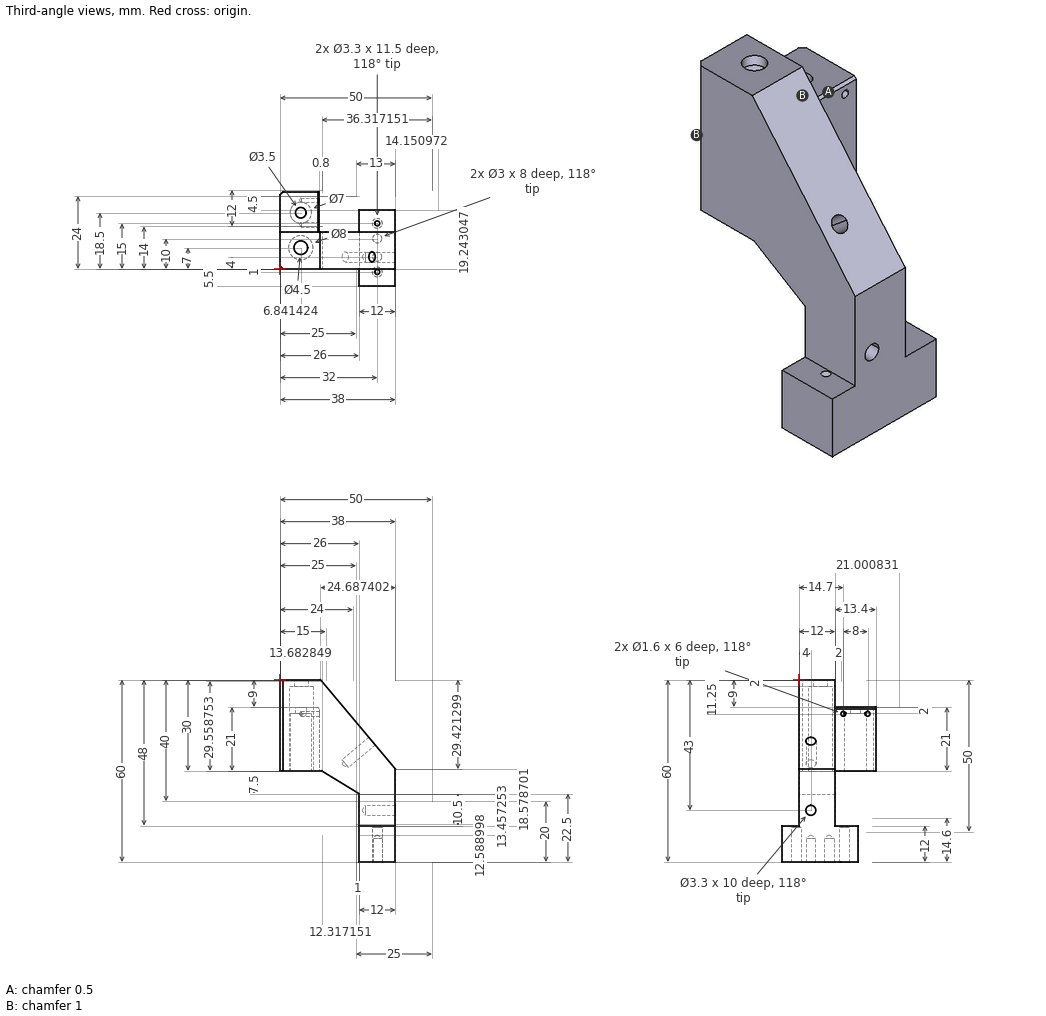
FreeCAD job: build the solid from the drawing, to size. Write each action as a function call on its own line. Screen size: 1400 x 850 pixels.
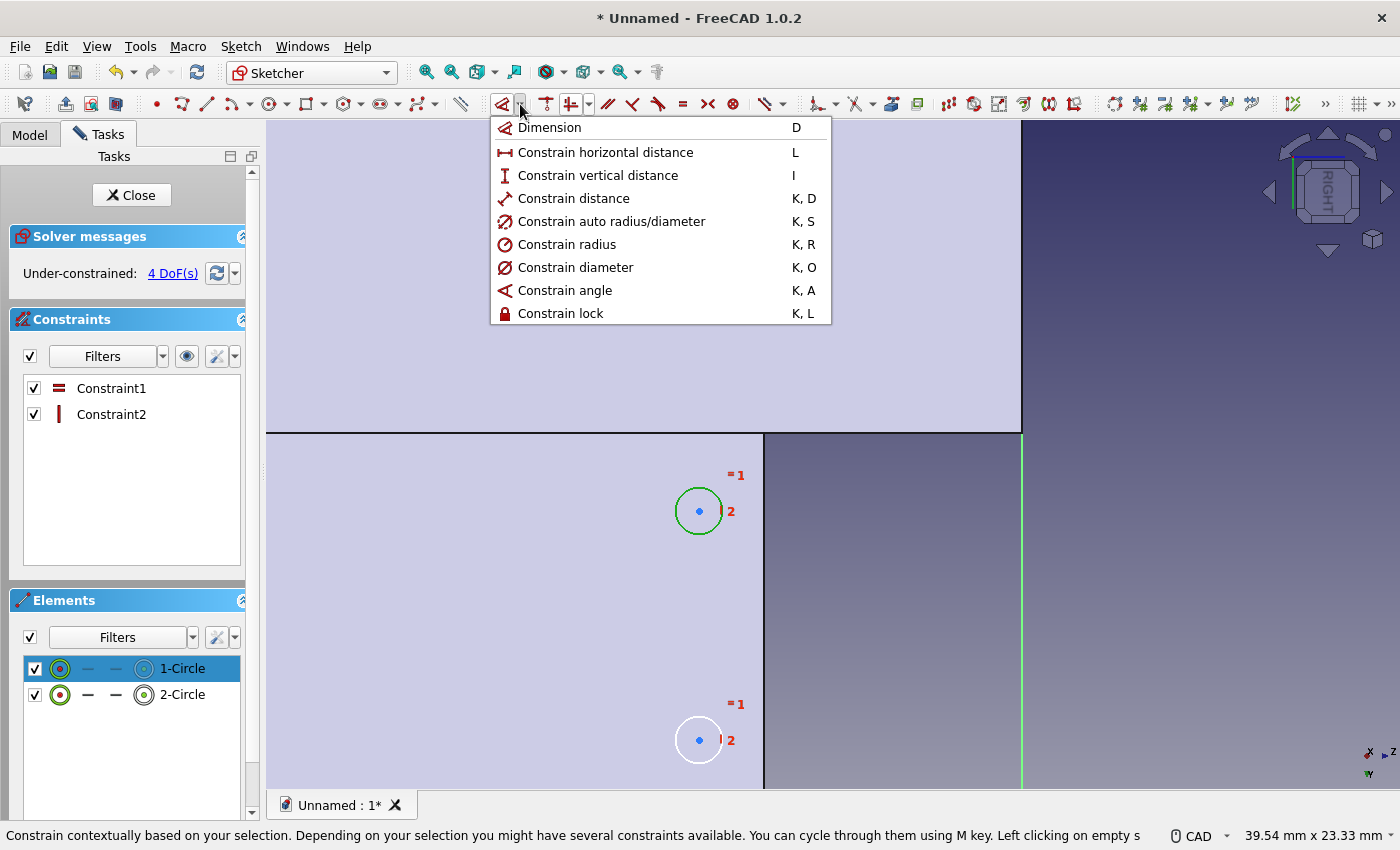
click(661, 268)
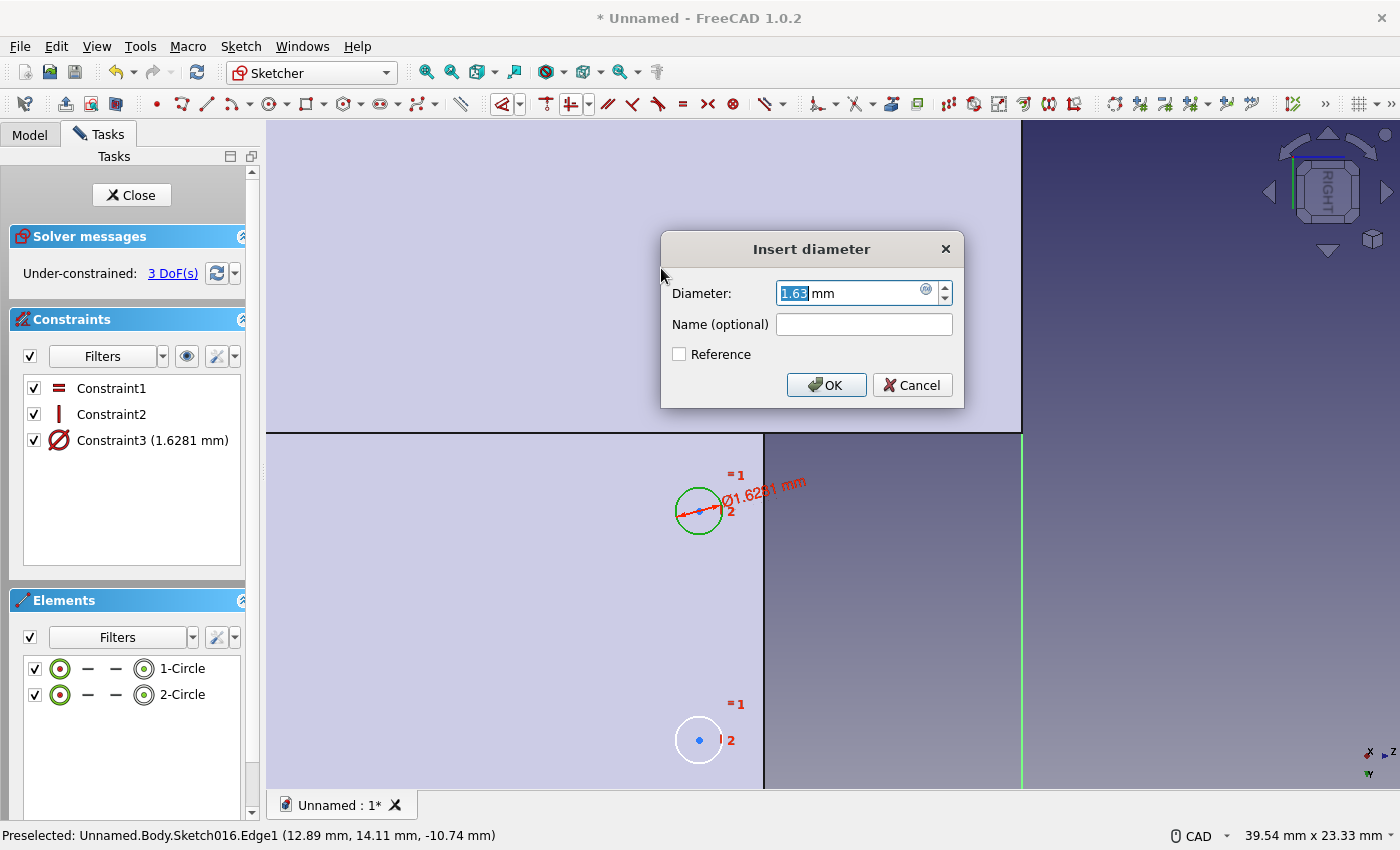
text(1.6)
key(Return)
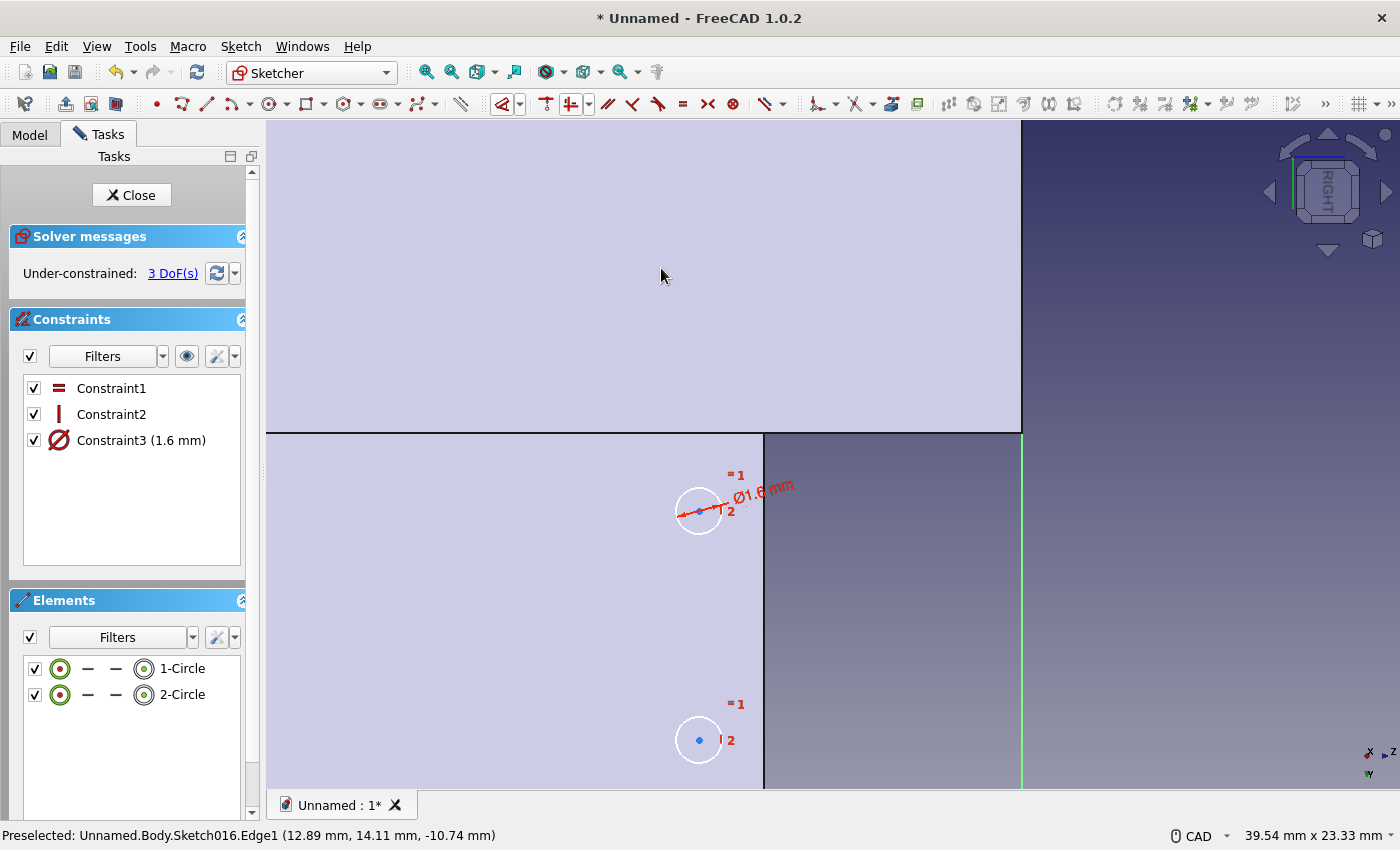
click(699, 511)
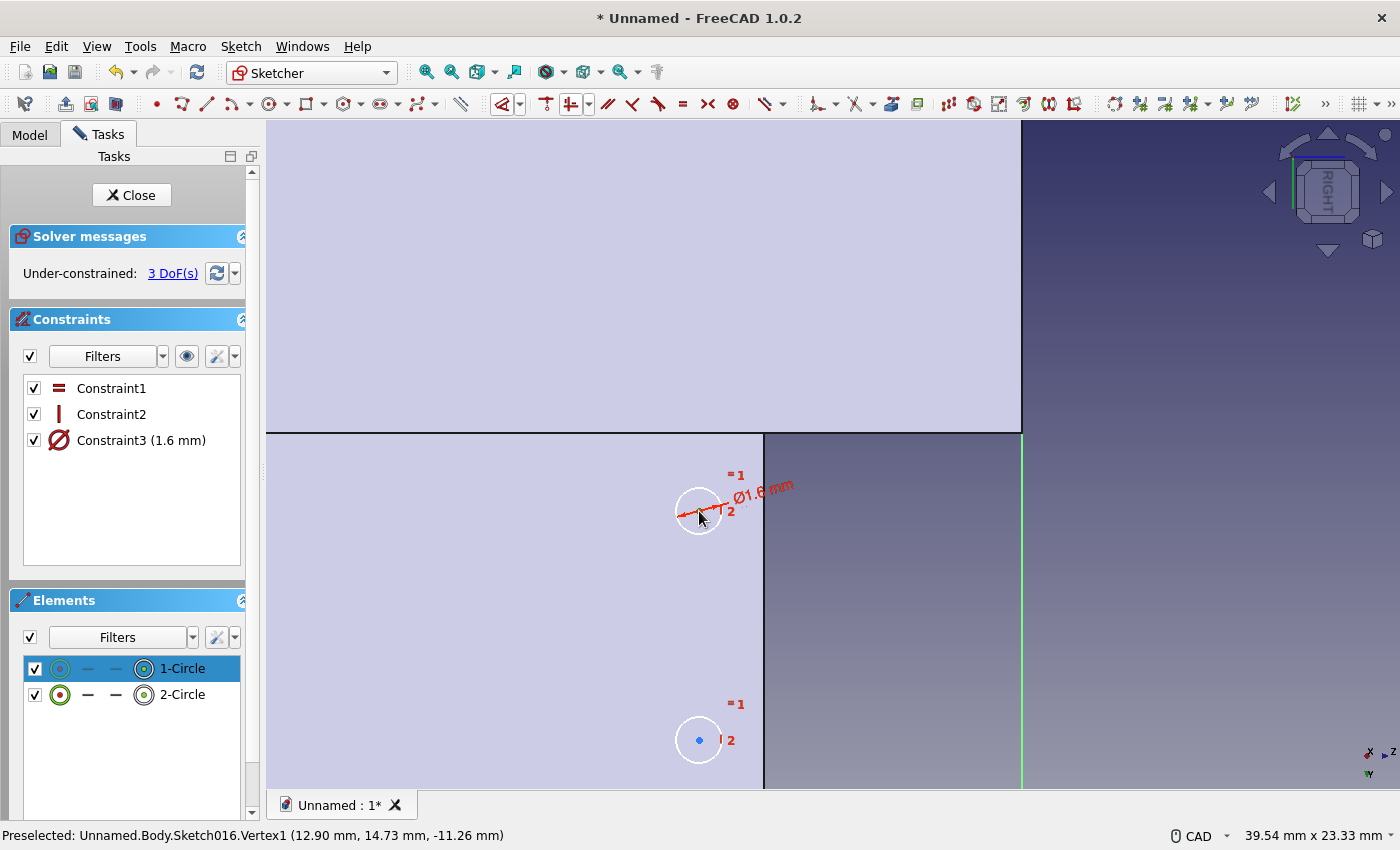
click(699, 740)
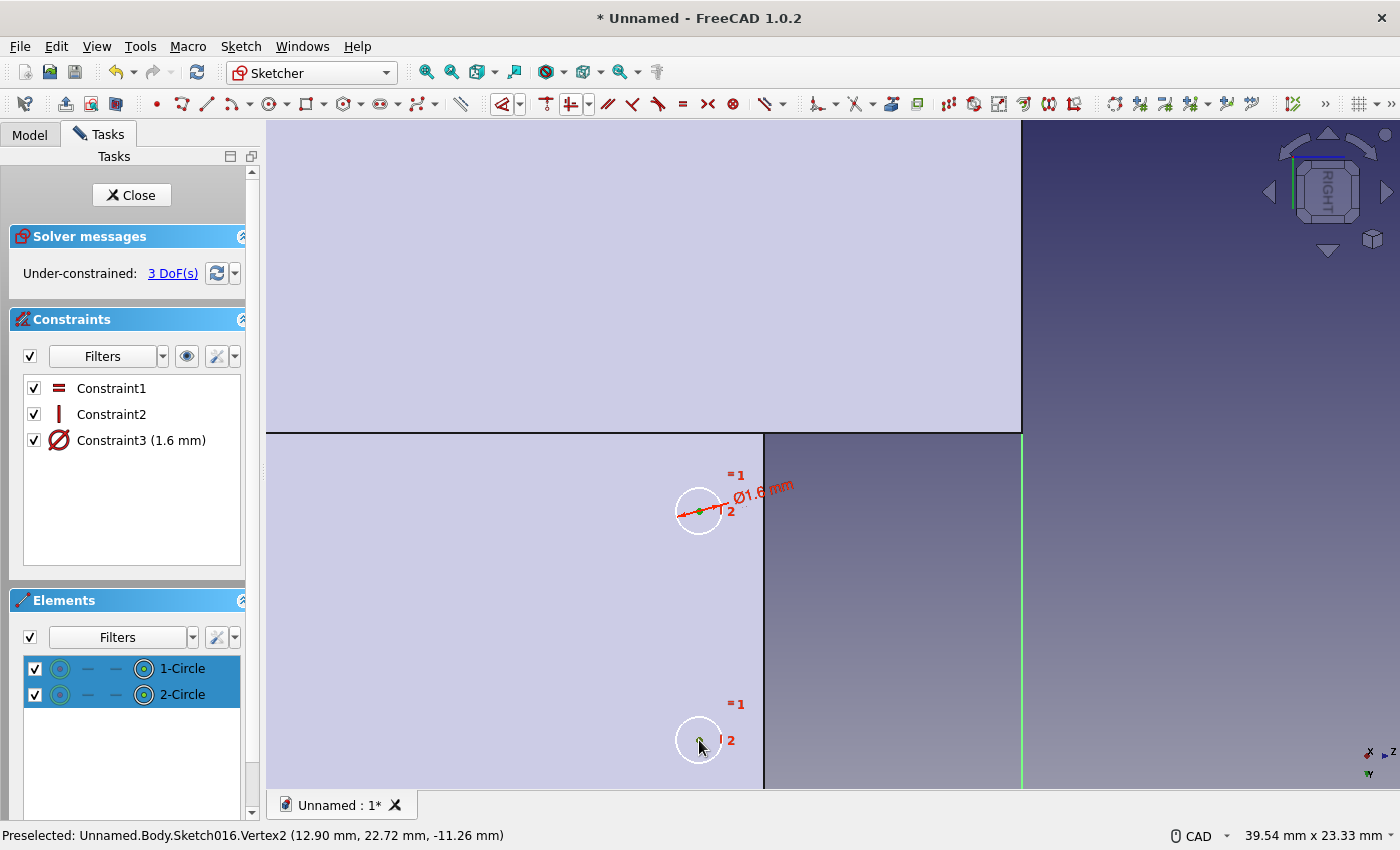
key(i)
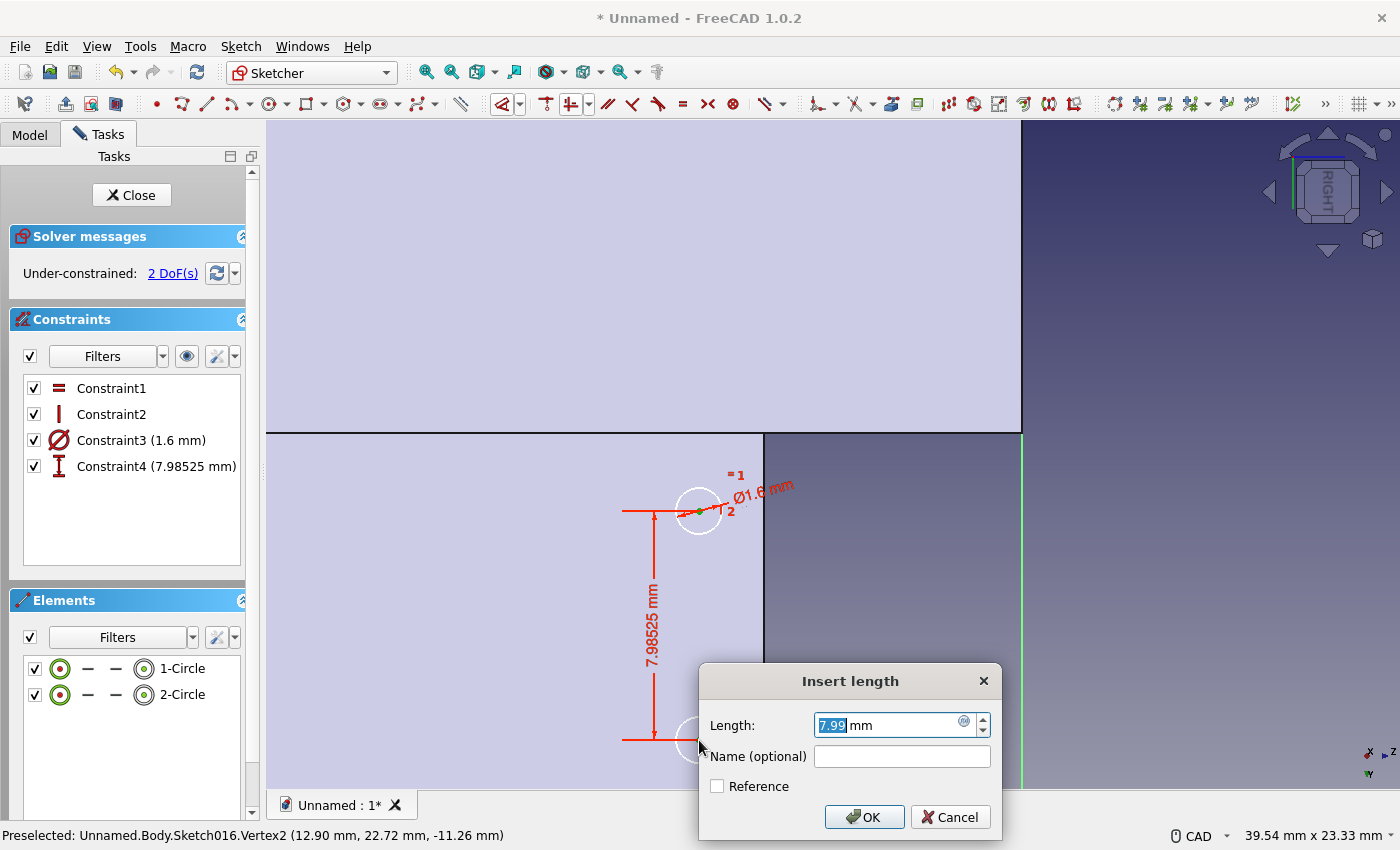
text(8)
key(Return)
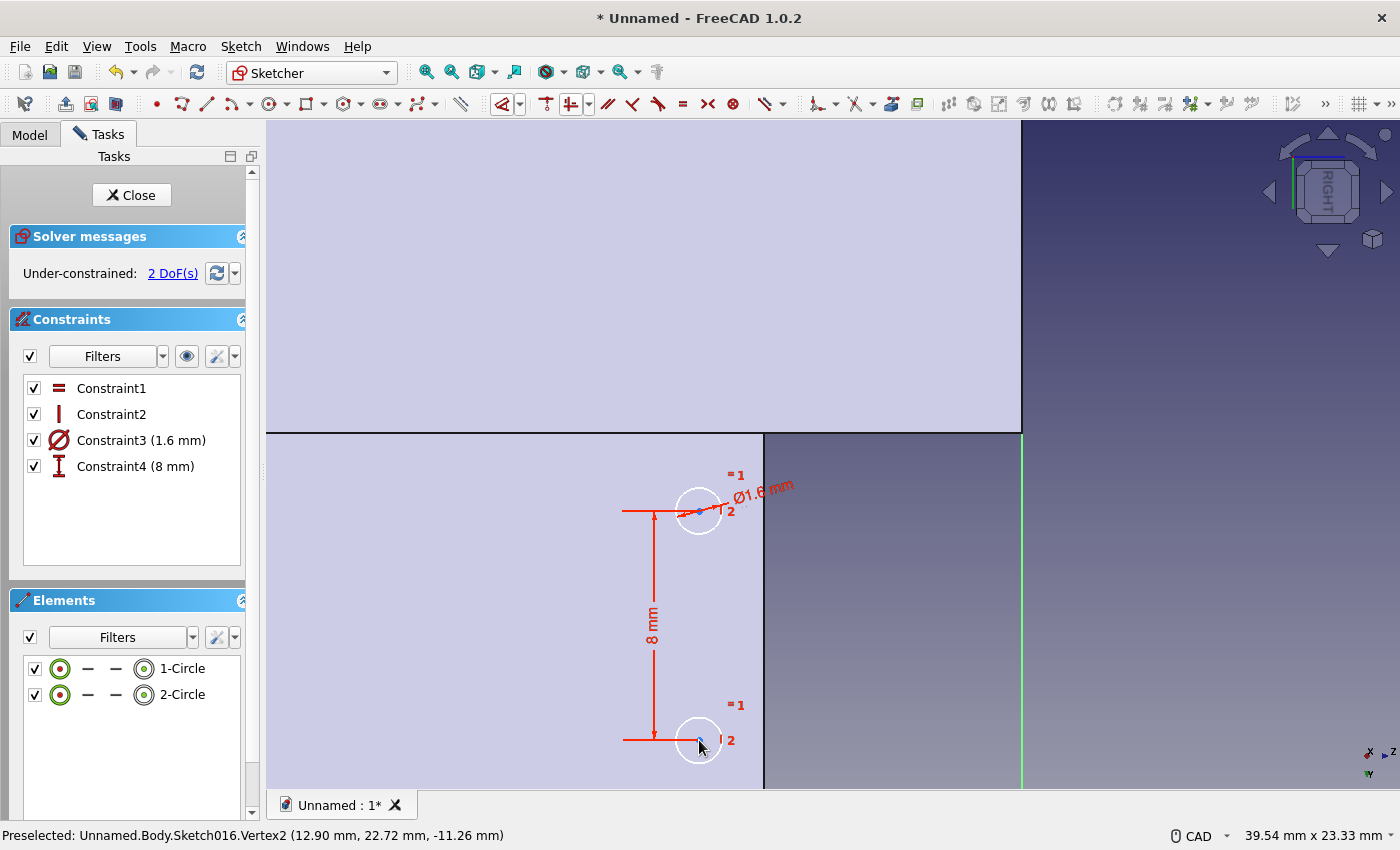
click(699, 511)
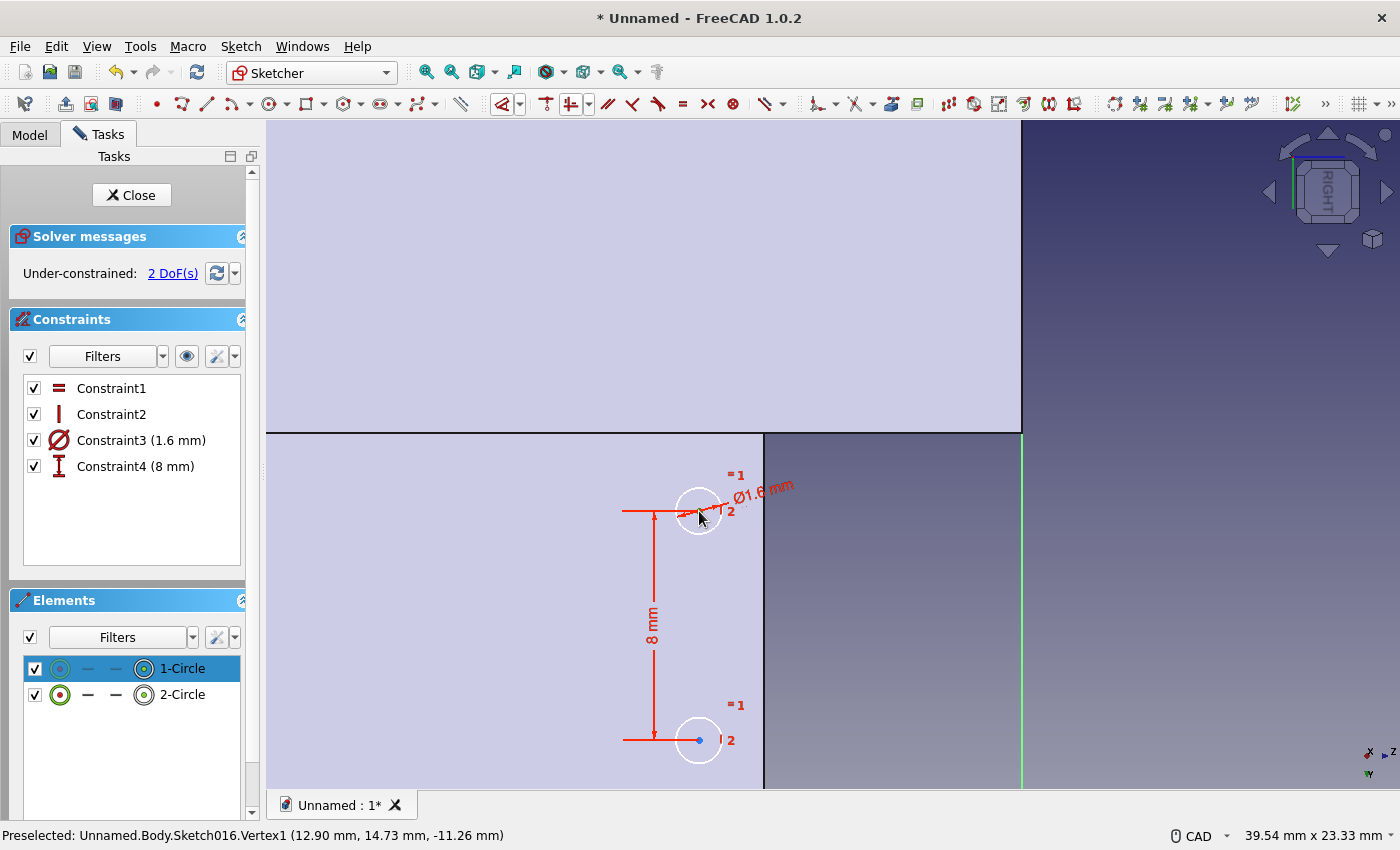
key(i)